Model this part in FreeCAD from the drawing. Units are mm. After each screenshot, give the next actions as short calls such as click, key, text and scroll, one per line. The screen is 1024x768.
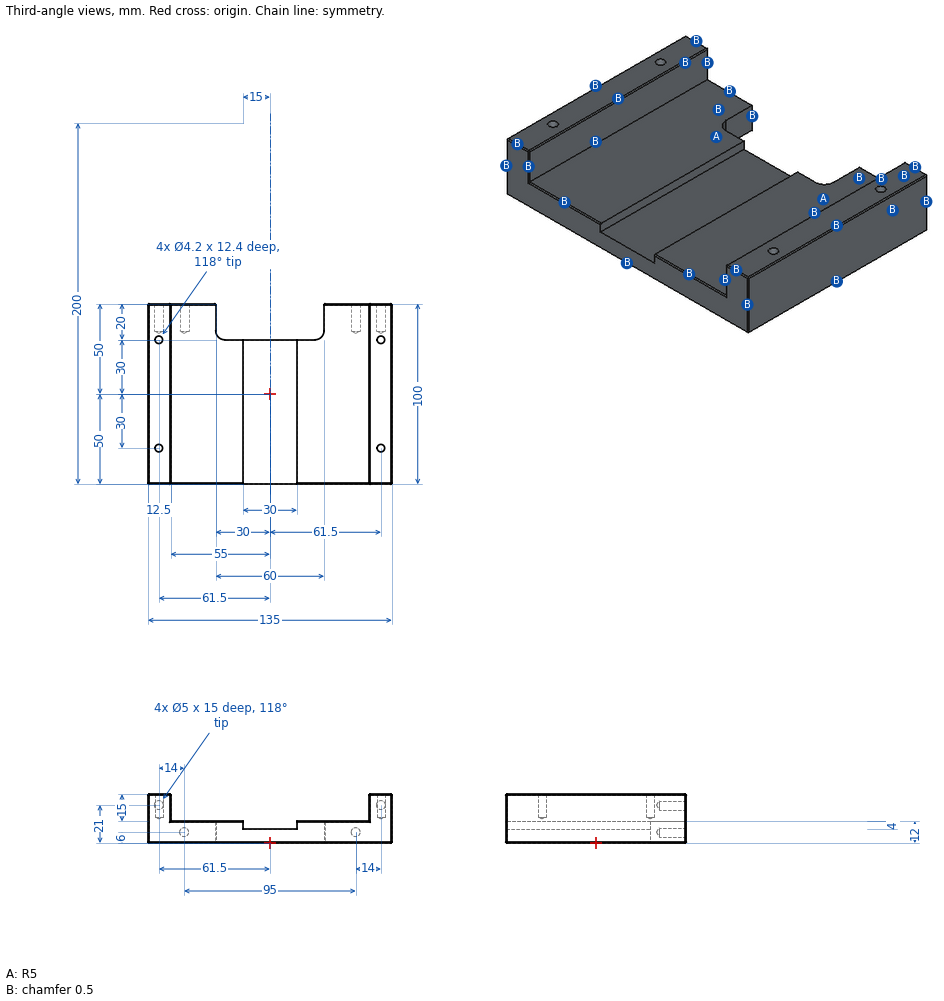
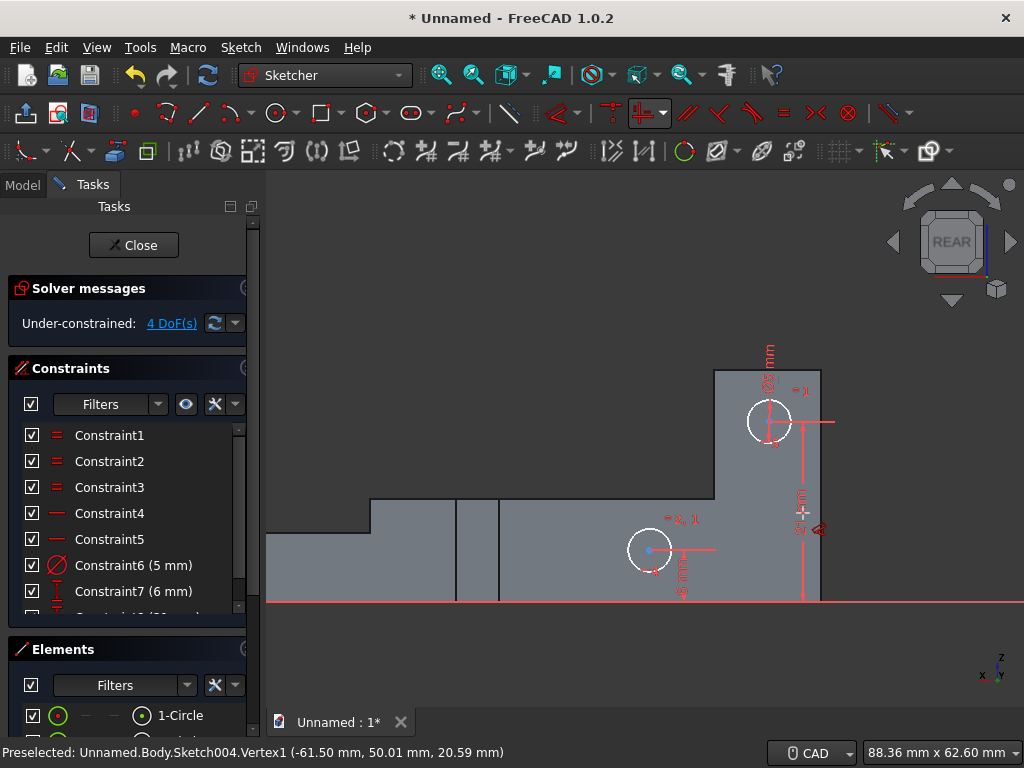
click(769, 422)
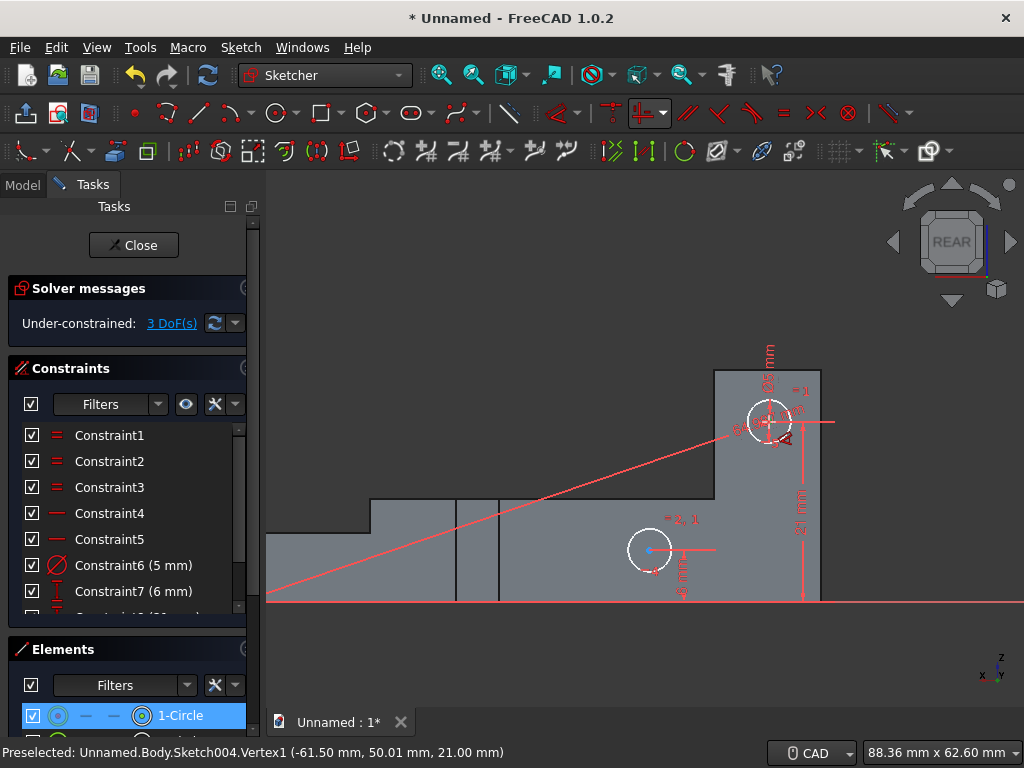
click(650, 550)
click(682, 388)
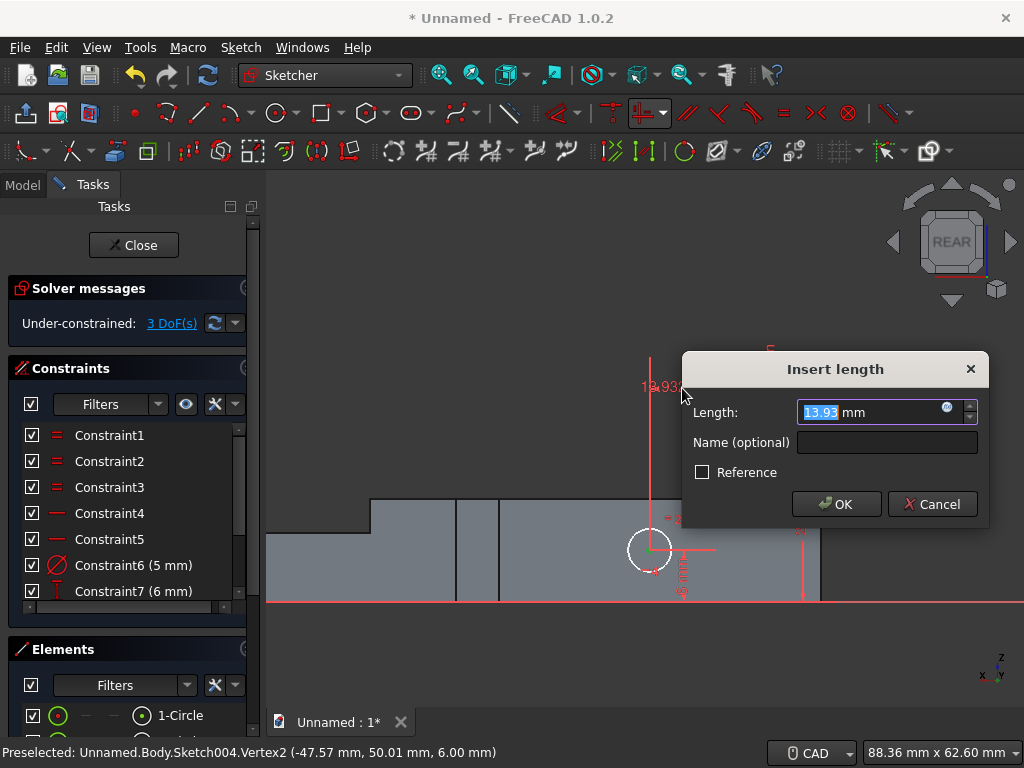
text(14)
key(Return)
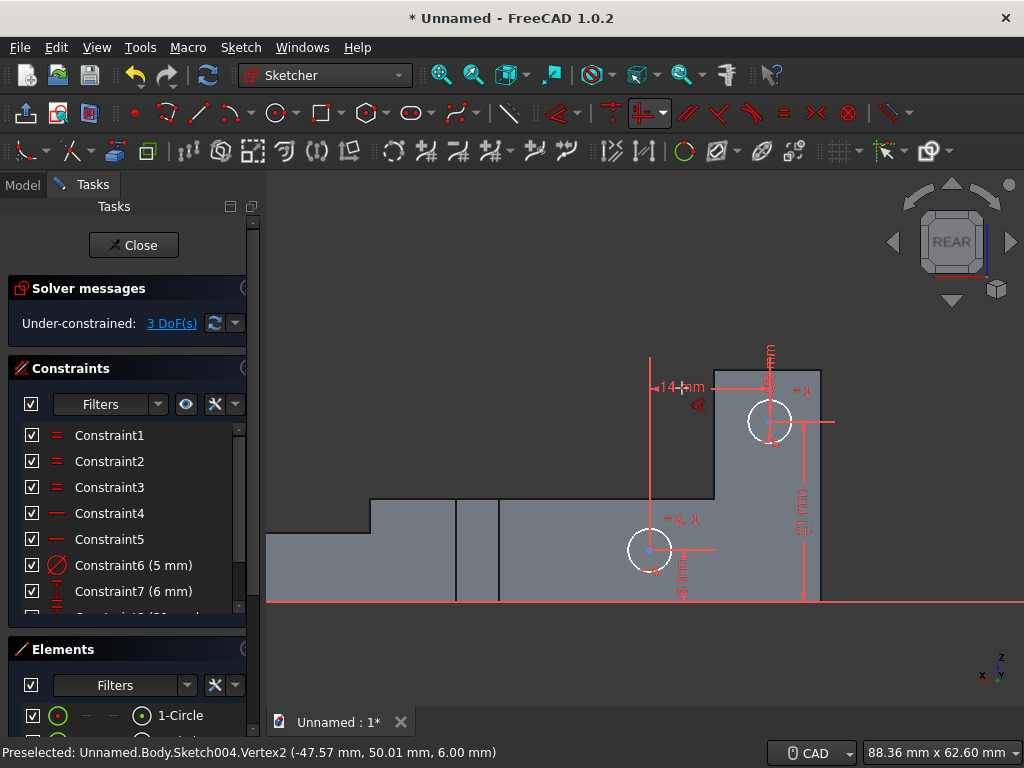
click(650, 550)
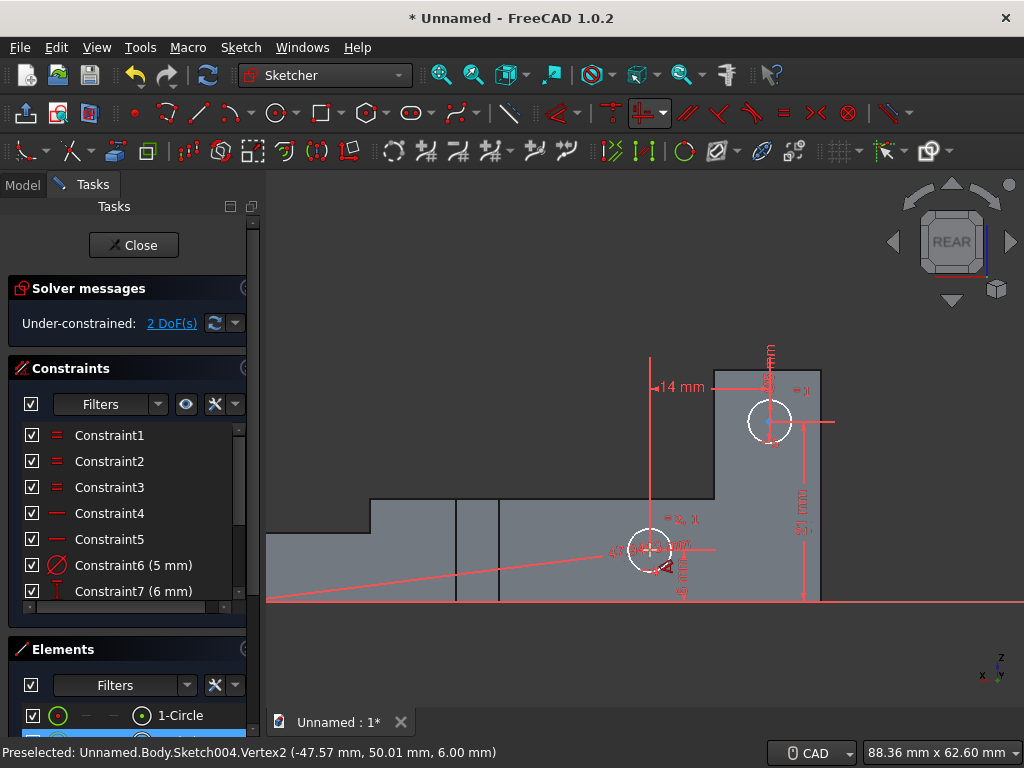
scroll(771, 402, down, 5)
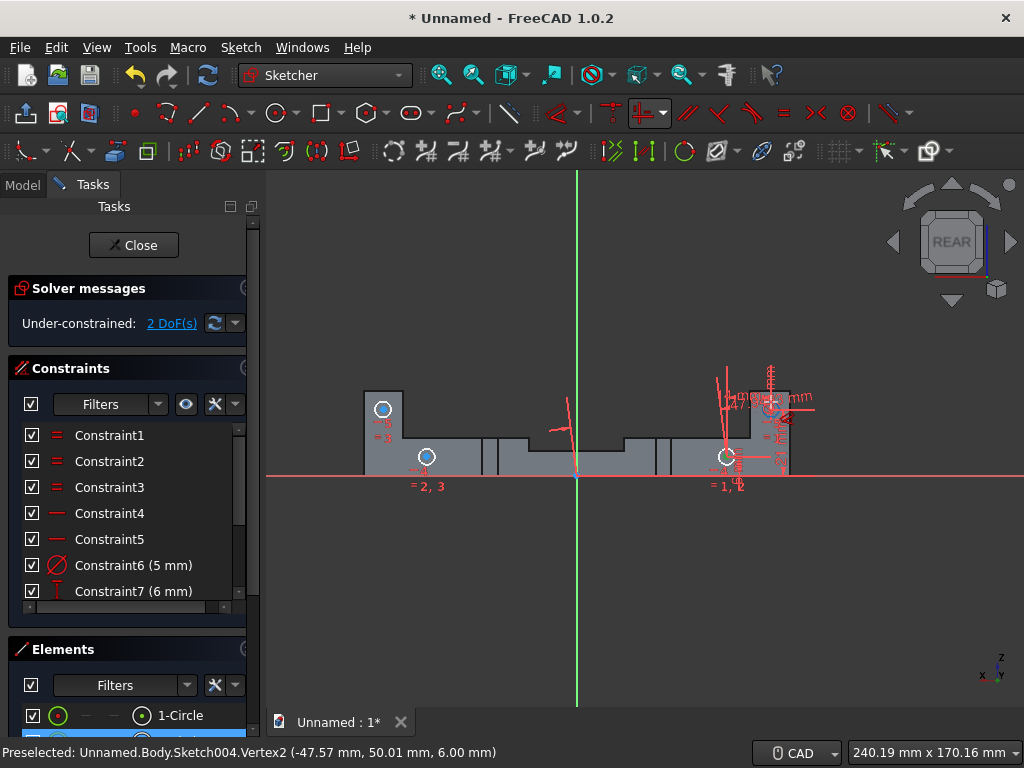
click(427, 457)
click(508, 491)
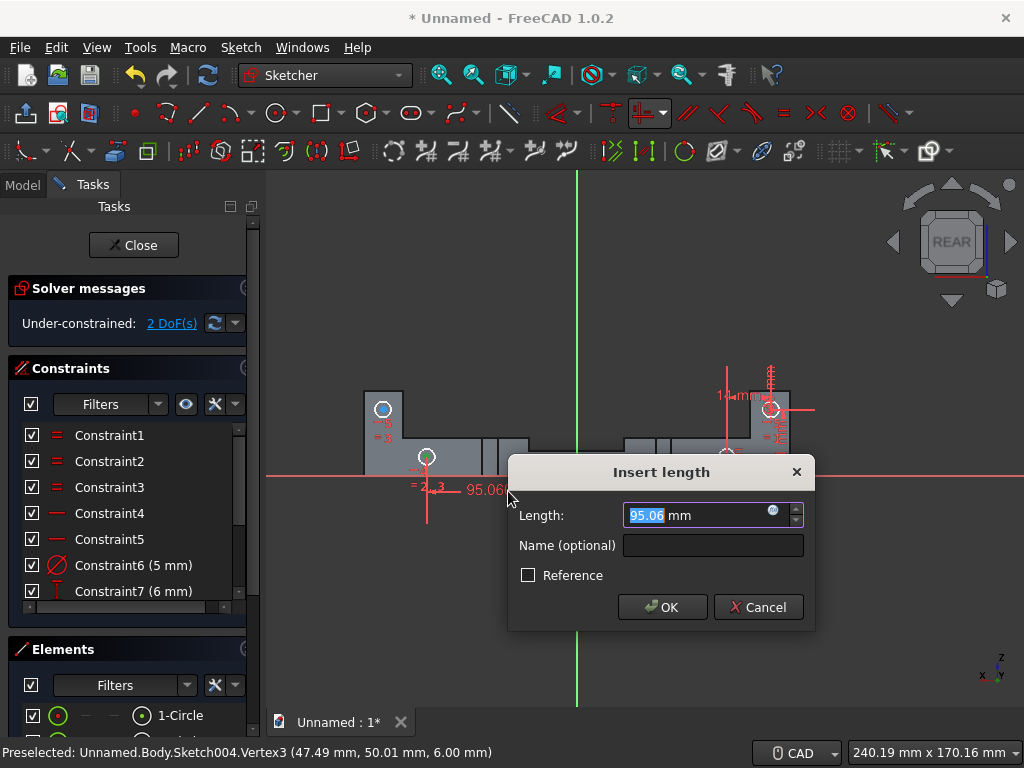
text(95)
key(Return)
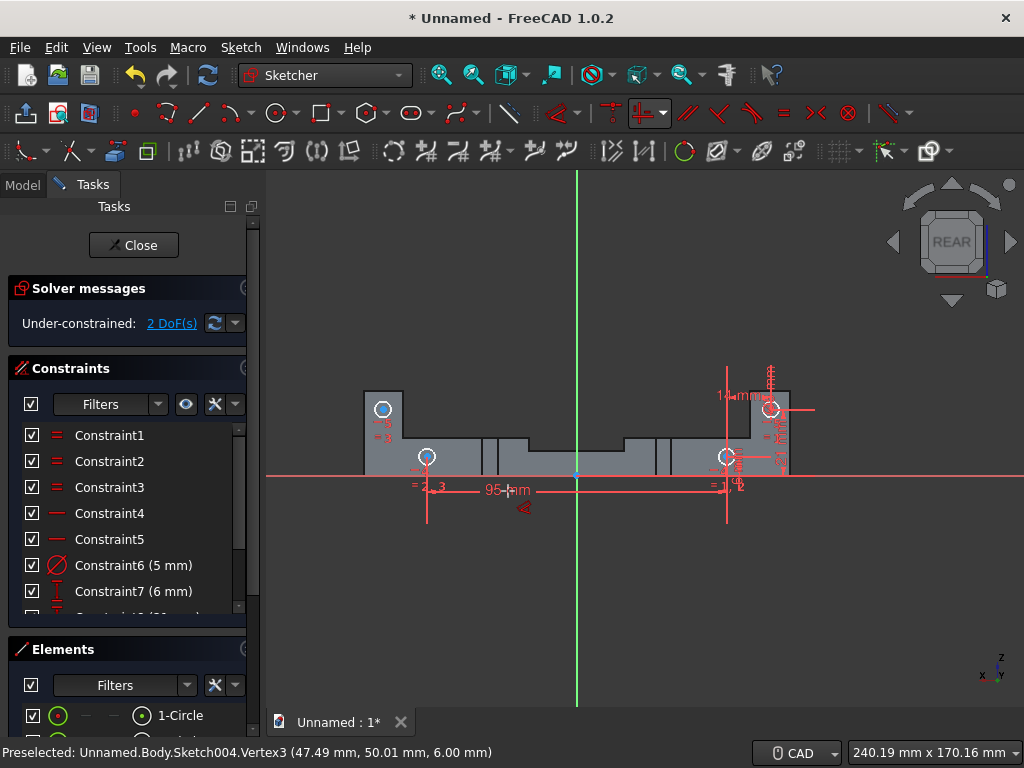
click(427, 457)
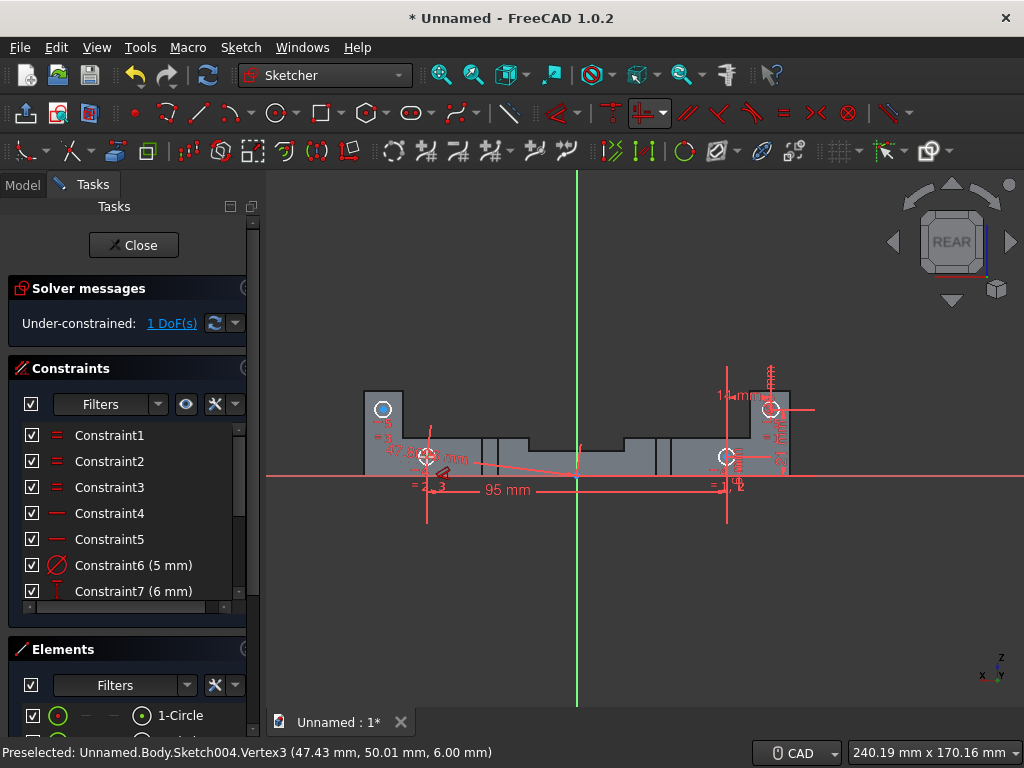
click(383, 409)
click(405, 375)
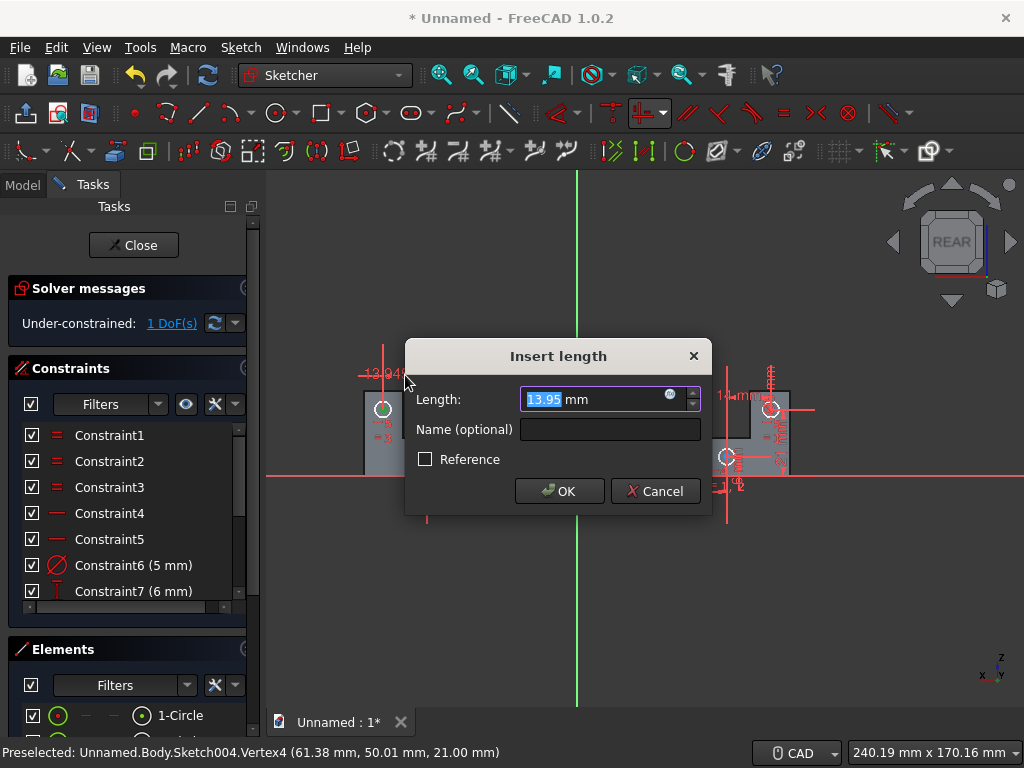
text(14)
key(Return)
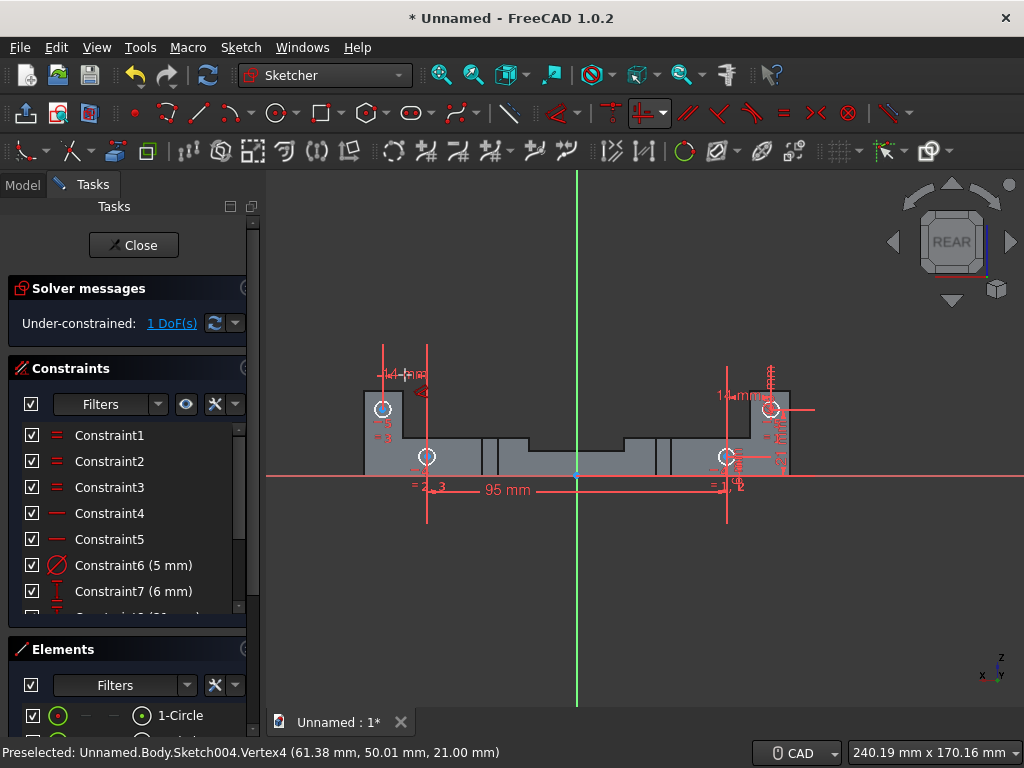
click(771, 409)
click(674, 510)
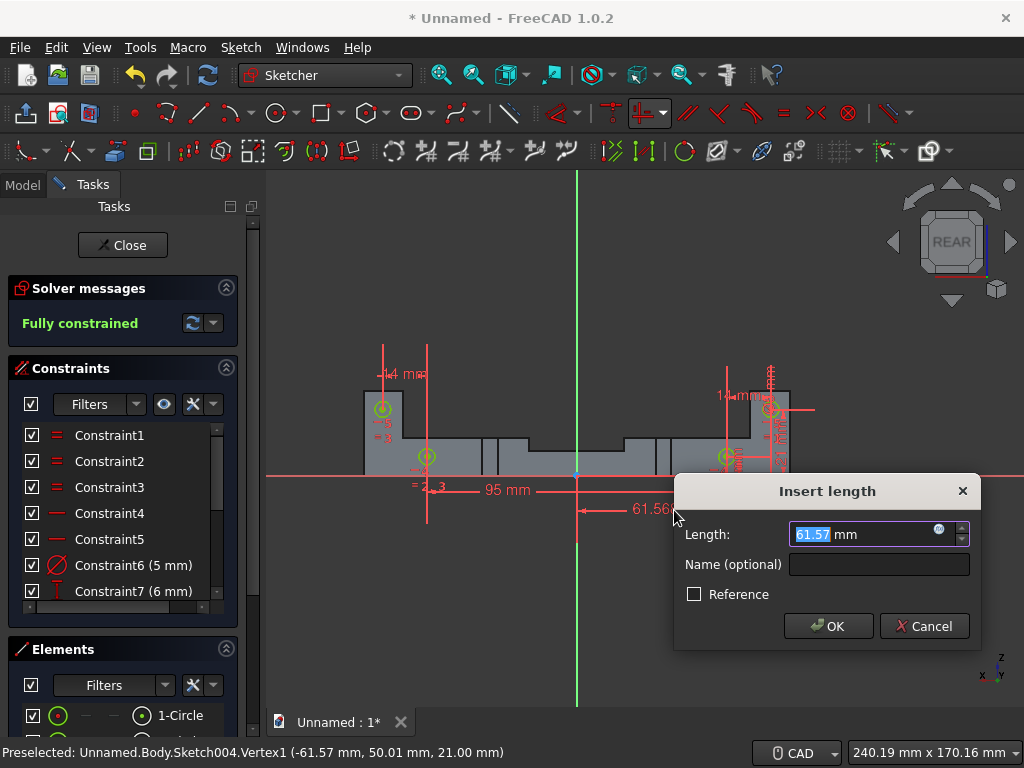
text(61.5)
key(Return)
key(Escape)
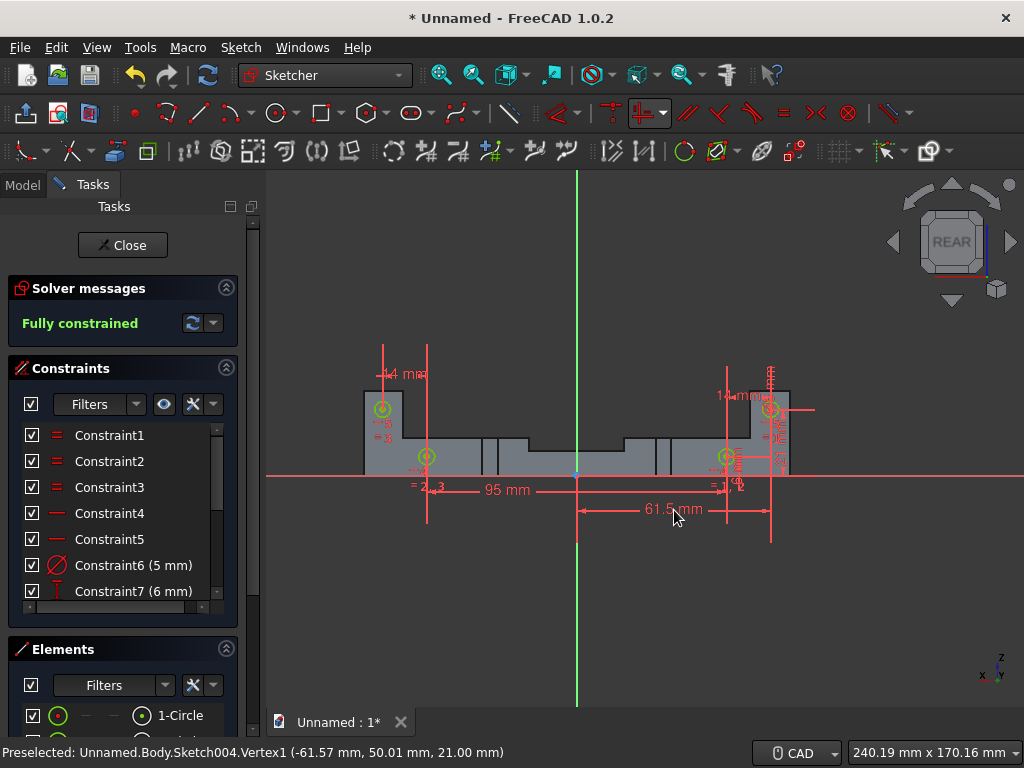
click(123, 245)